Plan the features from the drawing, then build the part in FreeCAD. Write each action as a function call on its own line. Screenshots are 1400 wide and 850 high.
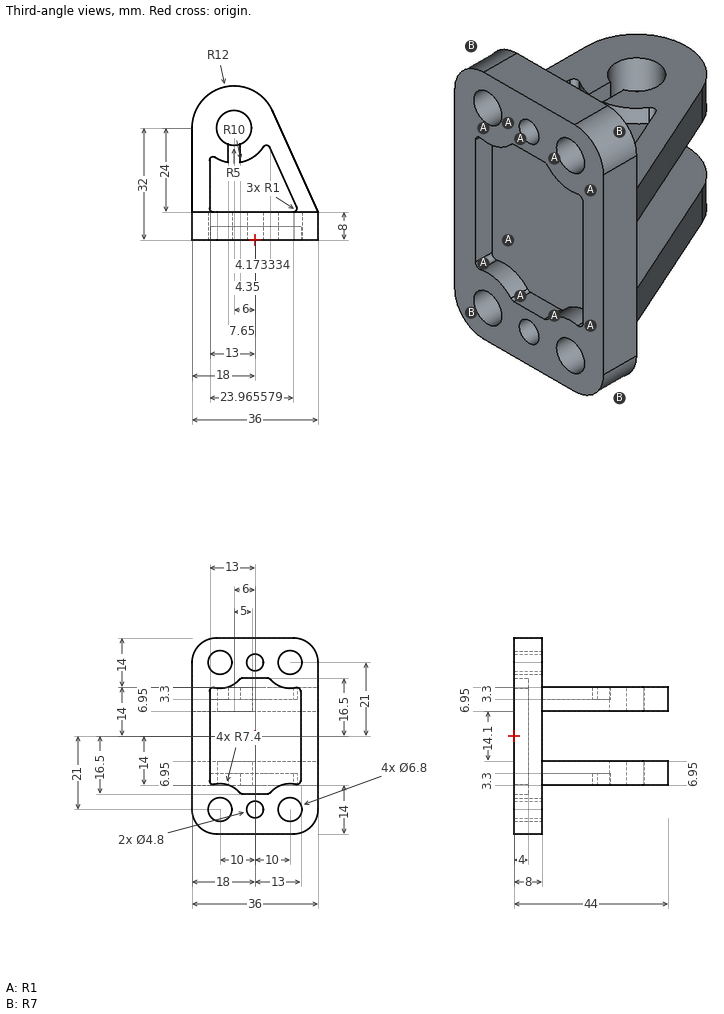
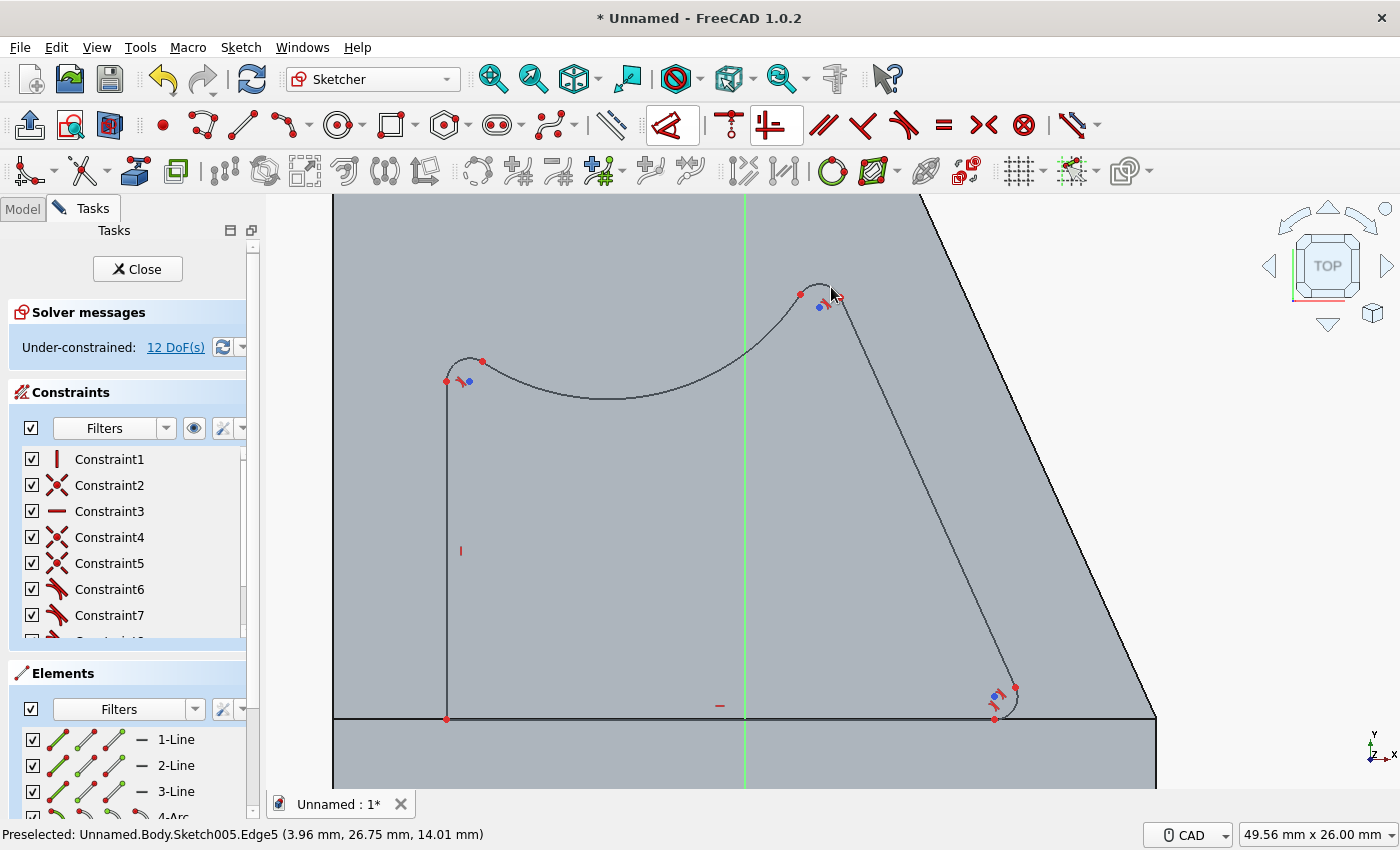
click(831, 287)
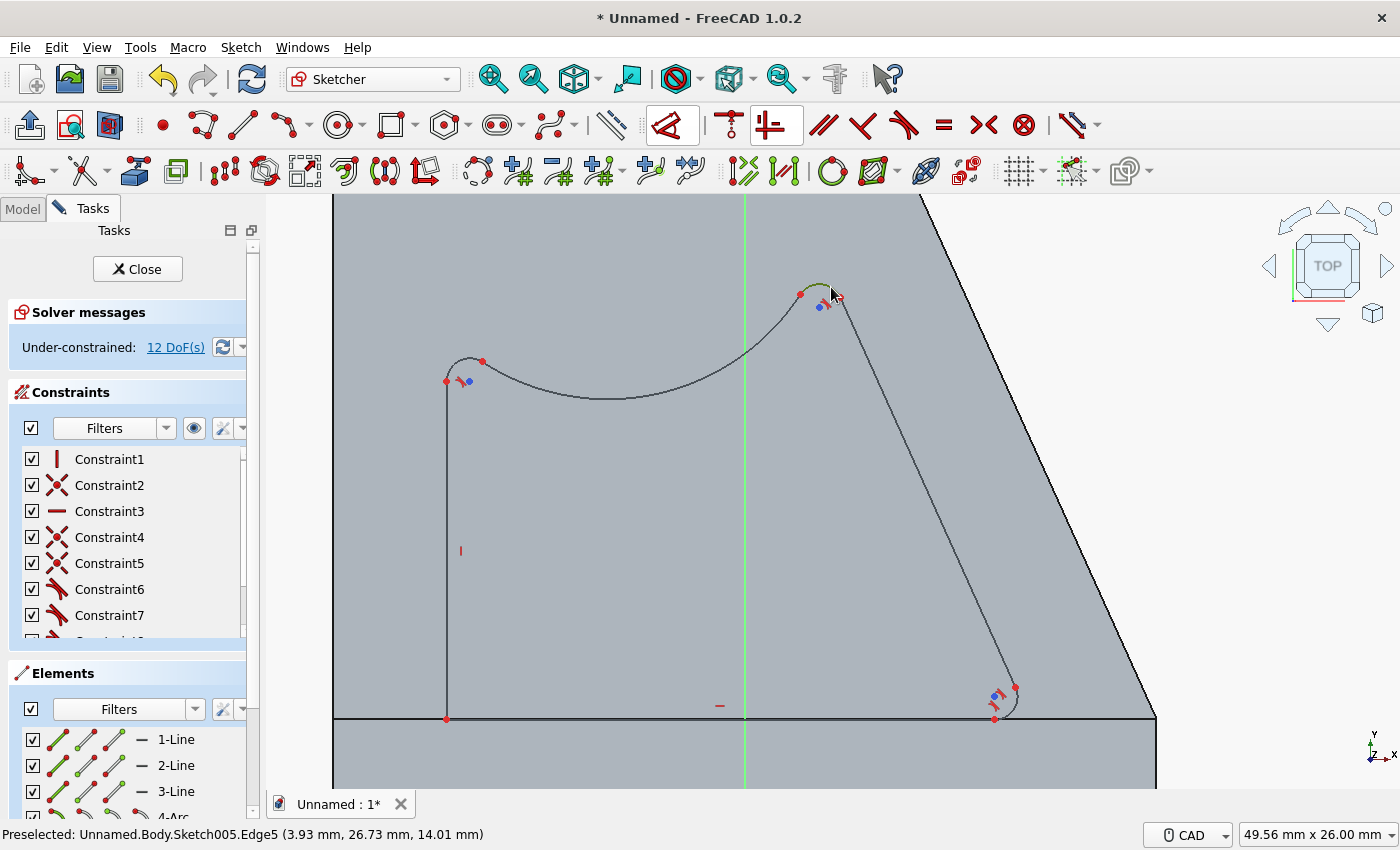
click(583, 398)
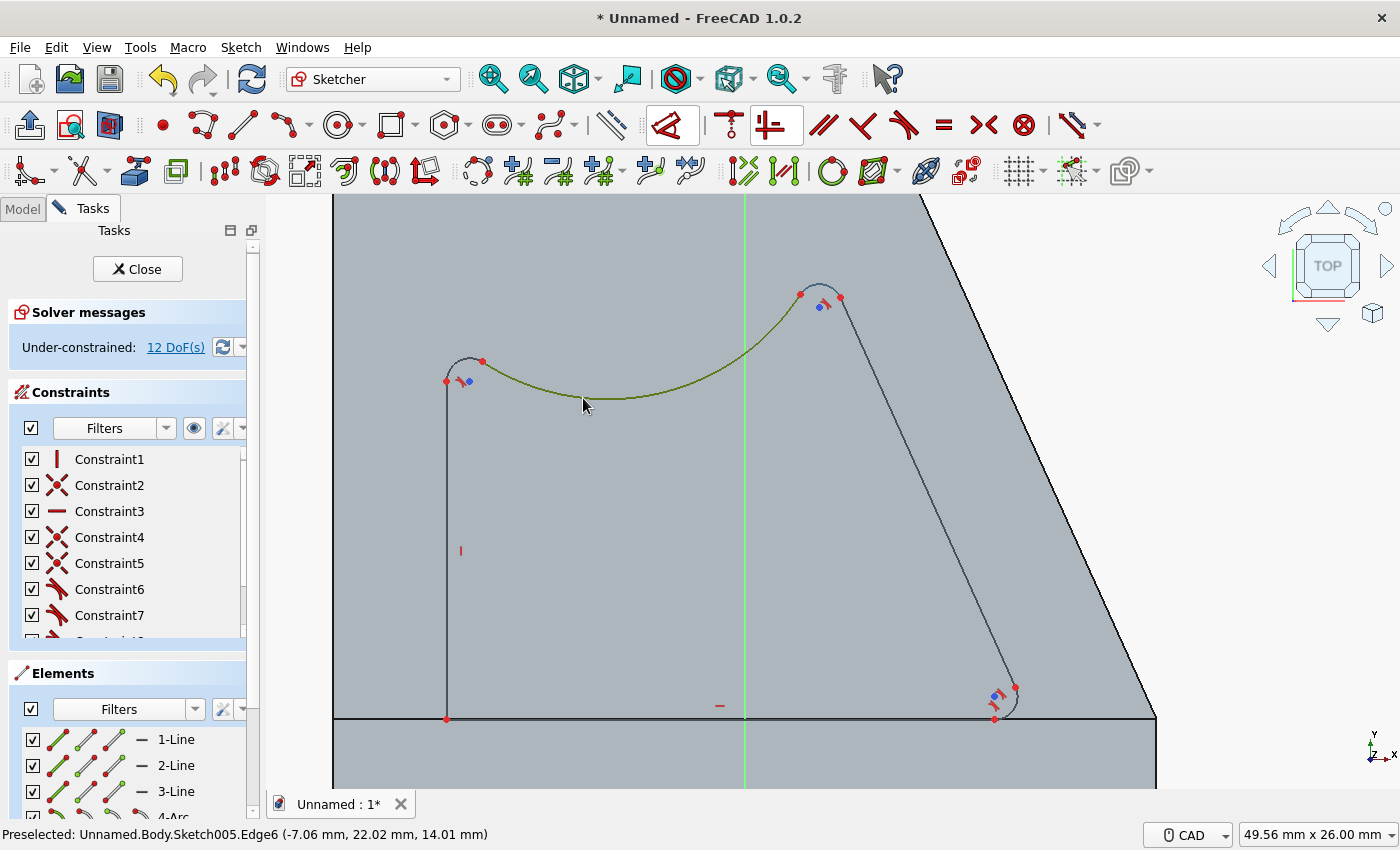
click(904, 126)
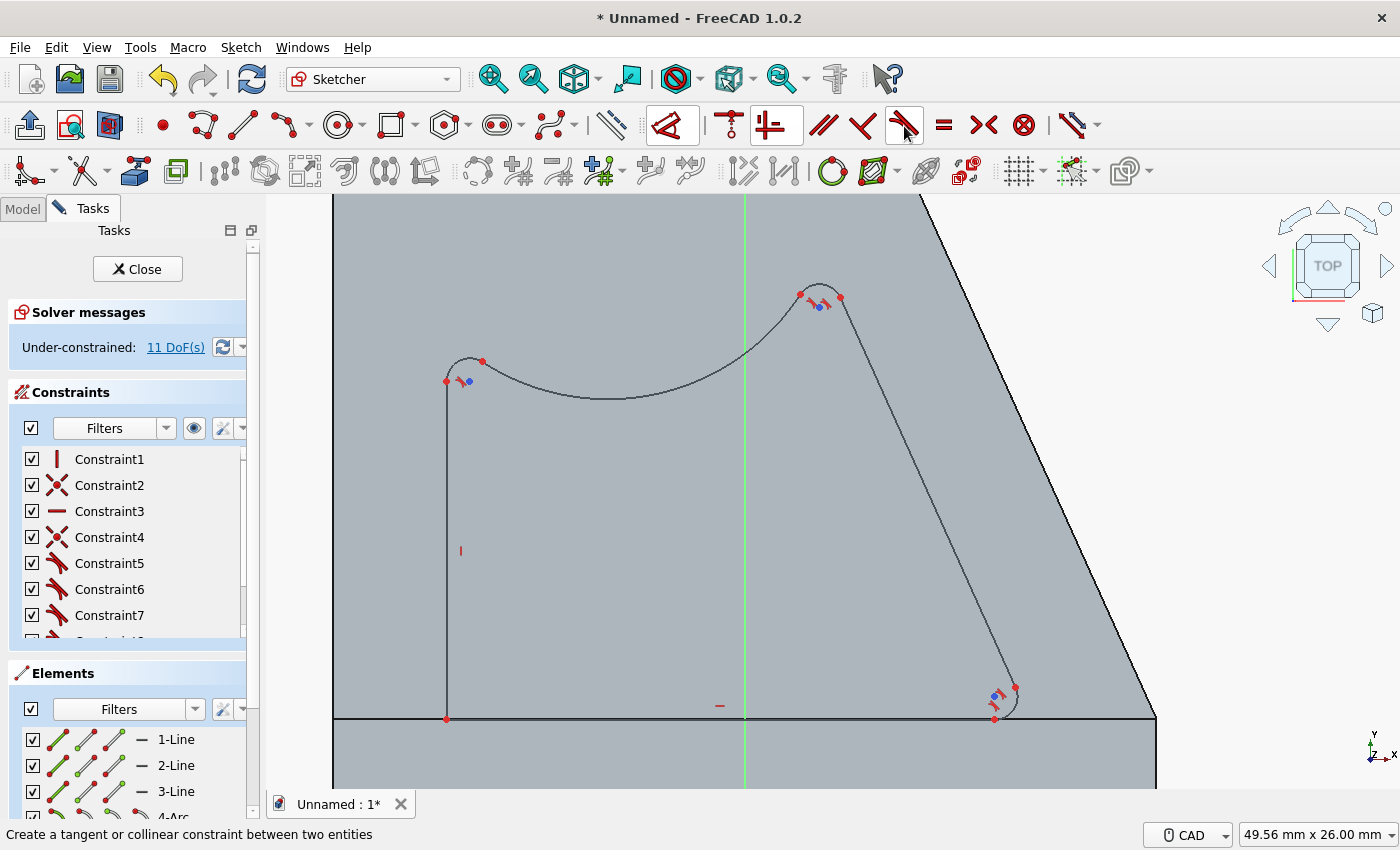
click(583, 398)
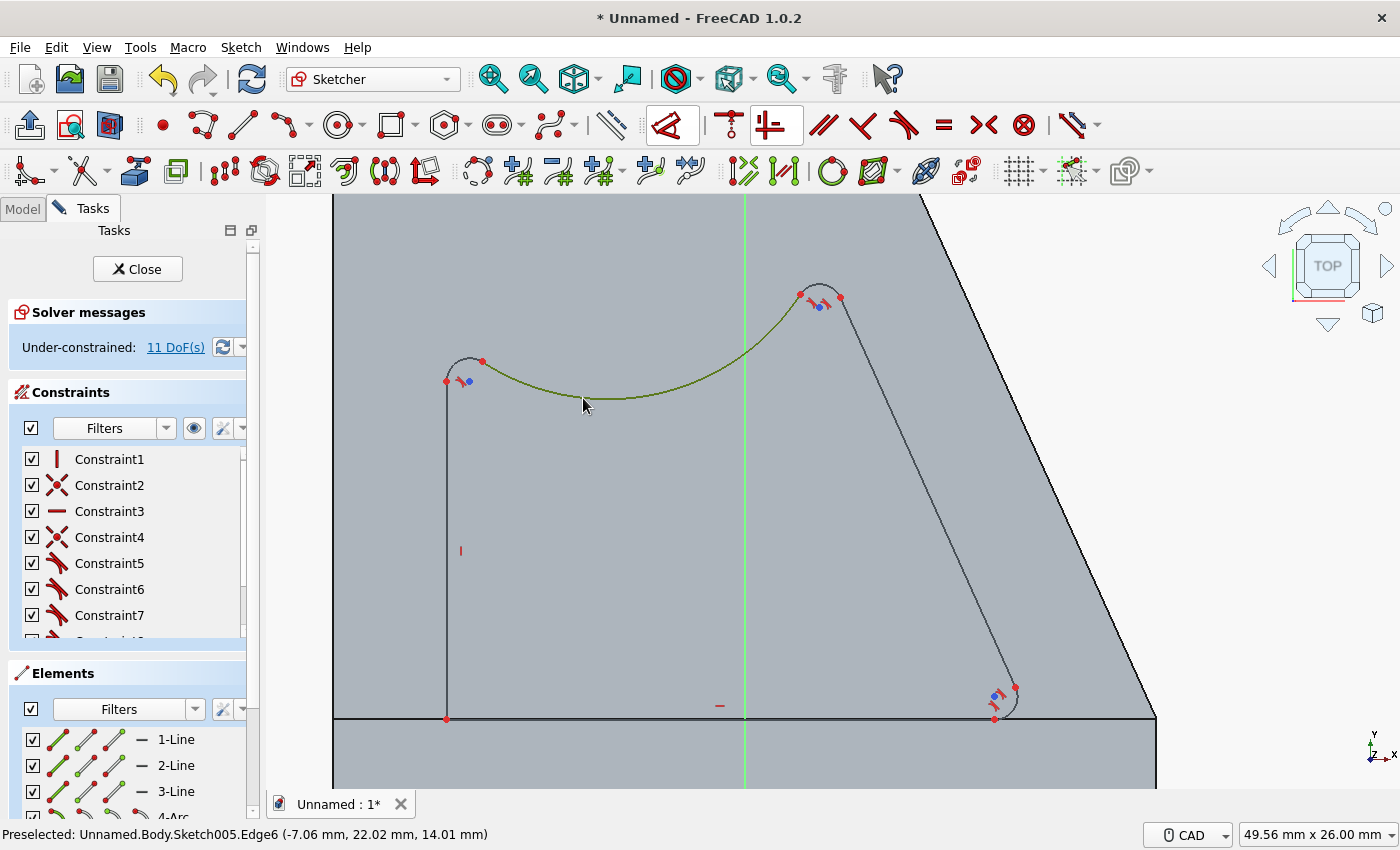
click(468, 358)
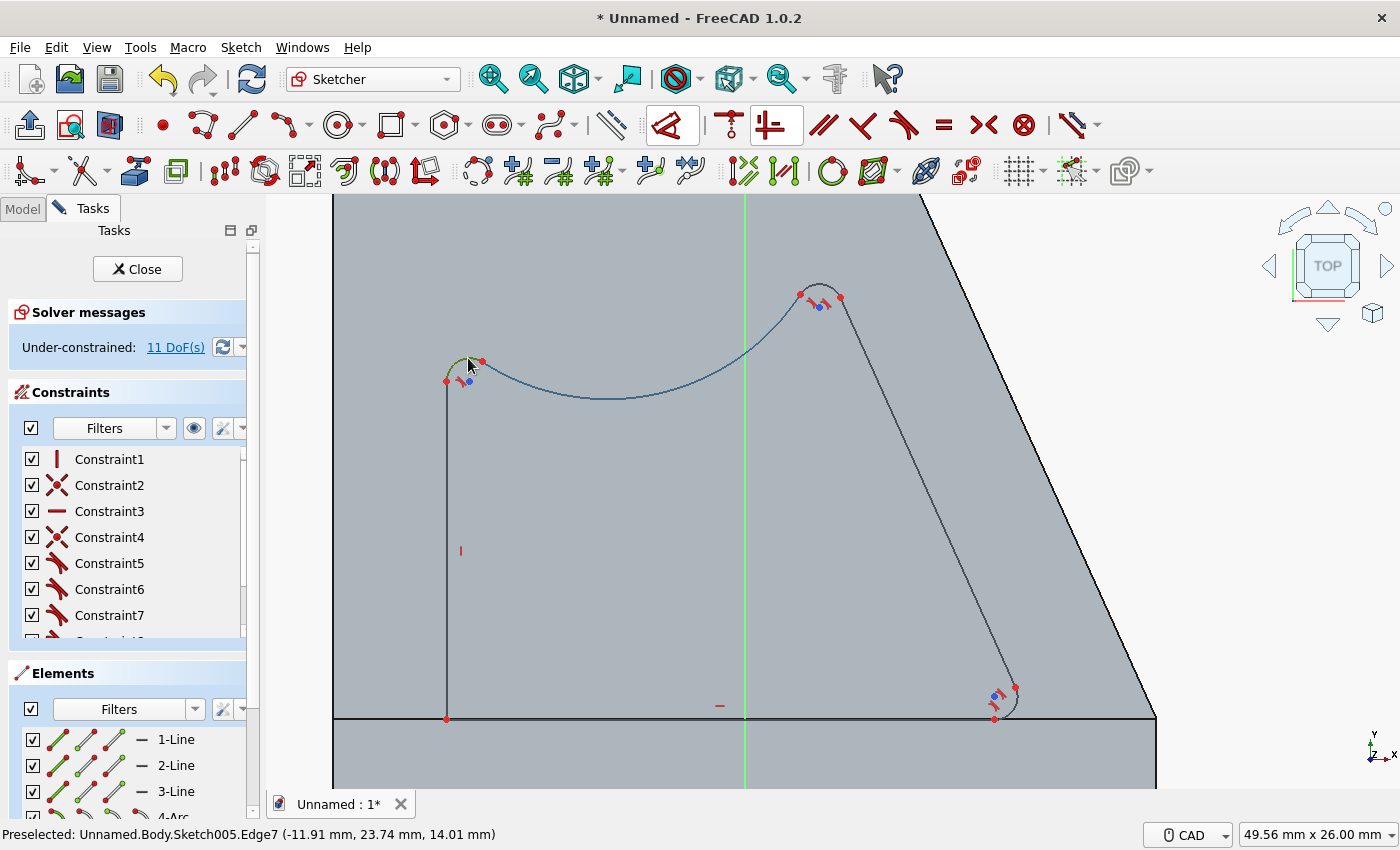
click(904, 126)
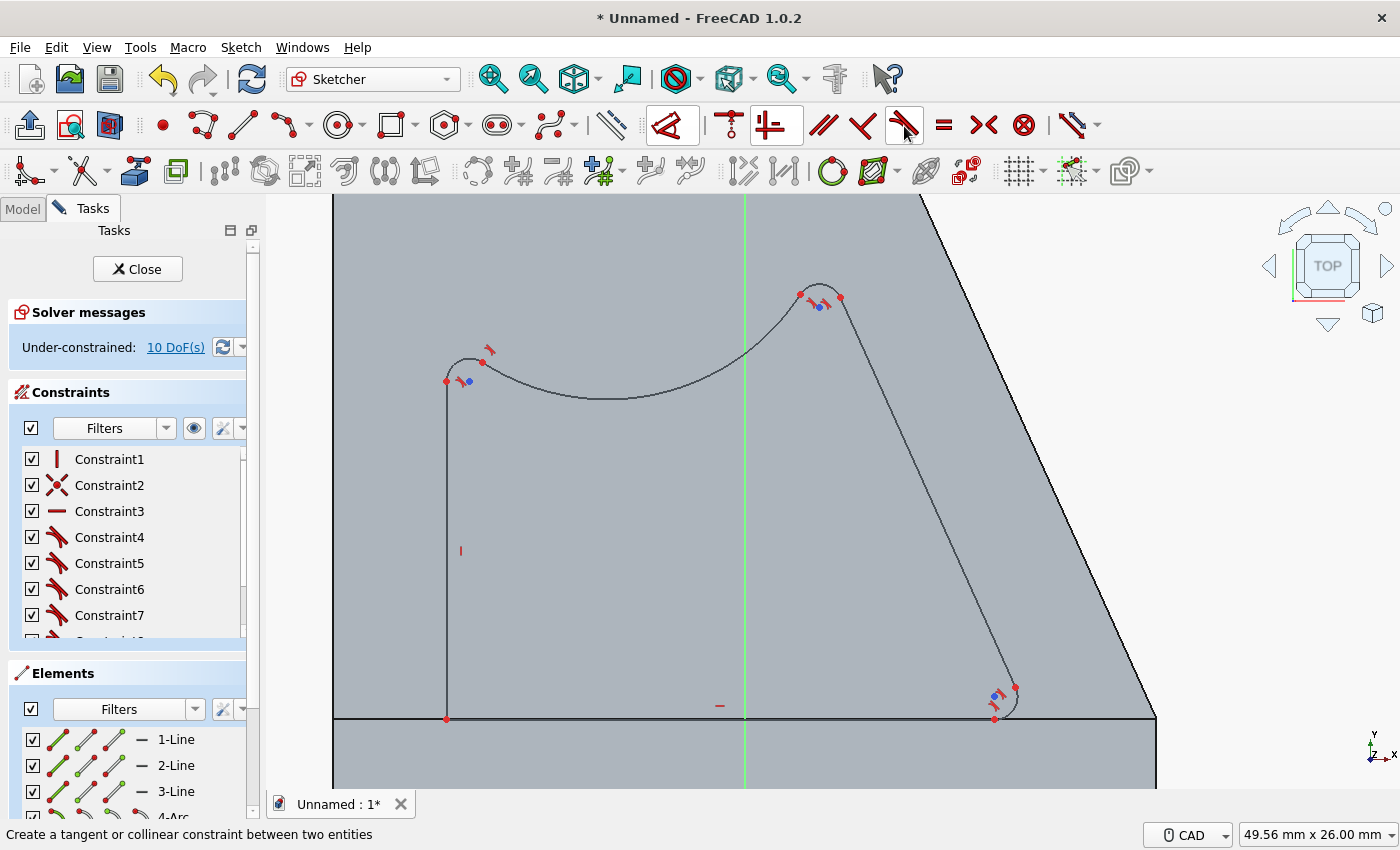
click(1007, 716)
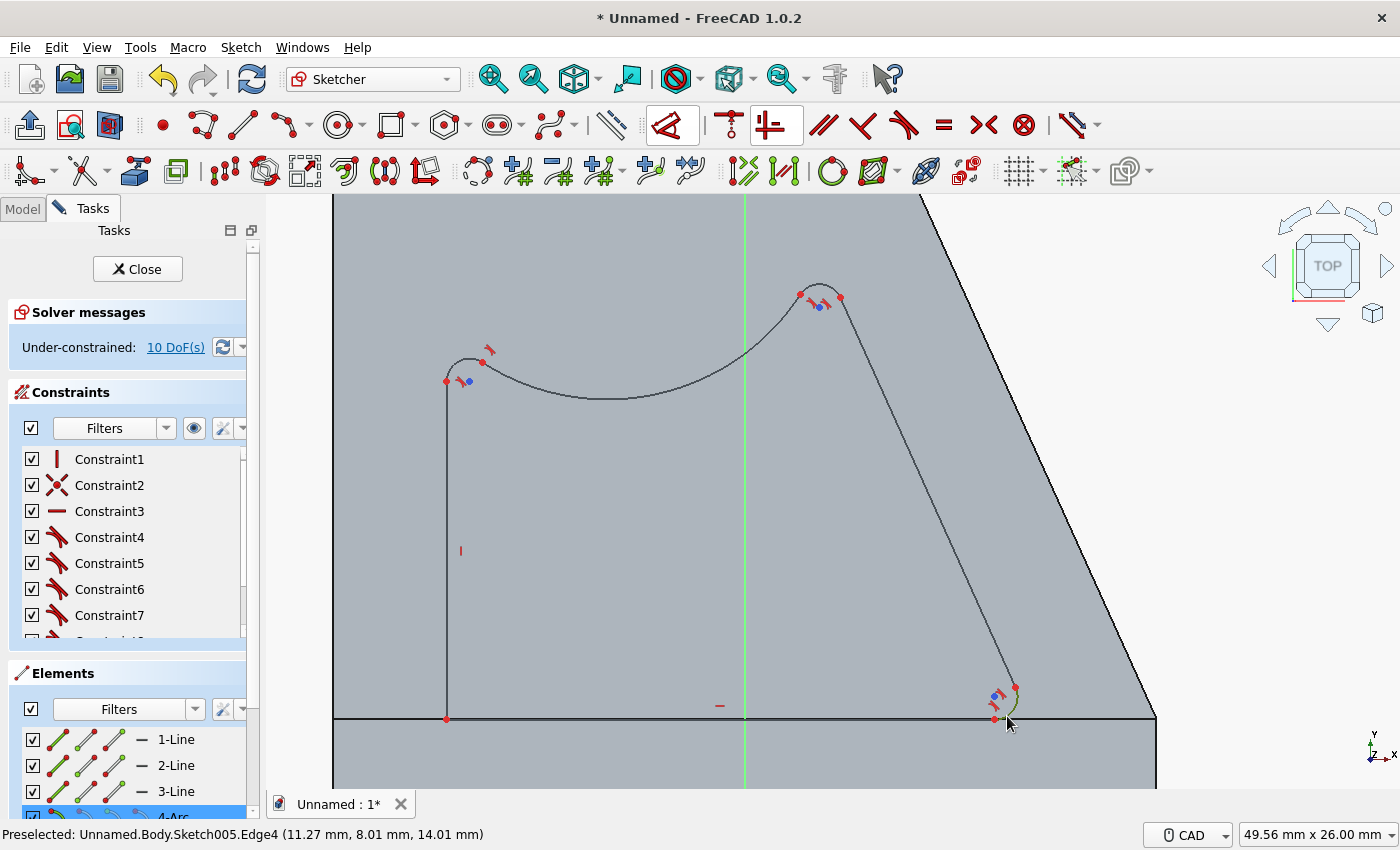
click(831, 287)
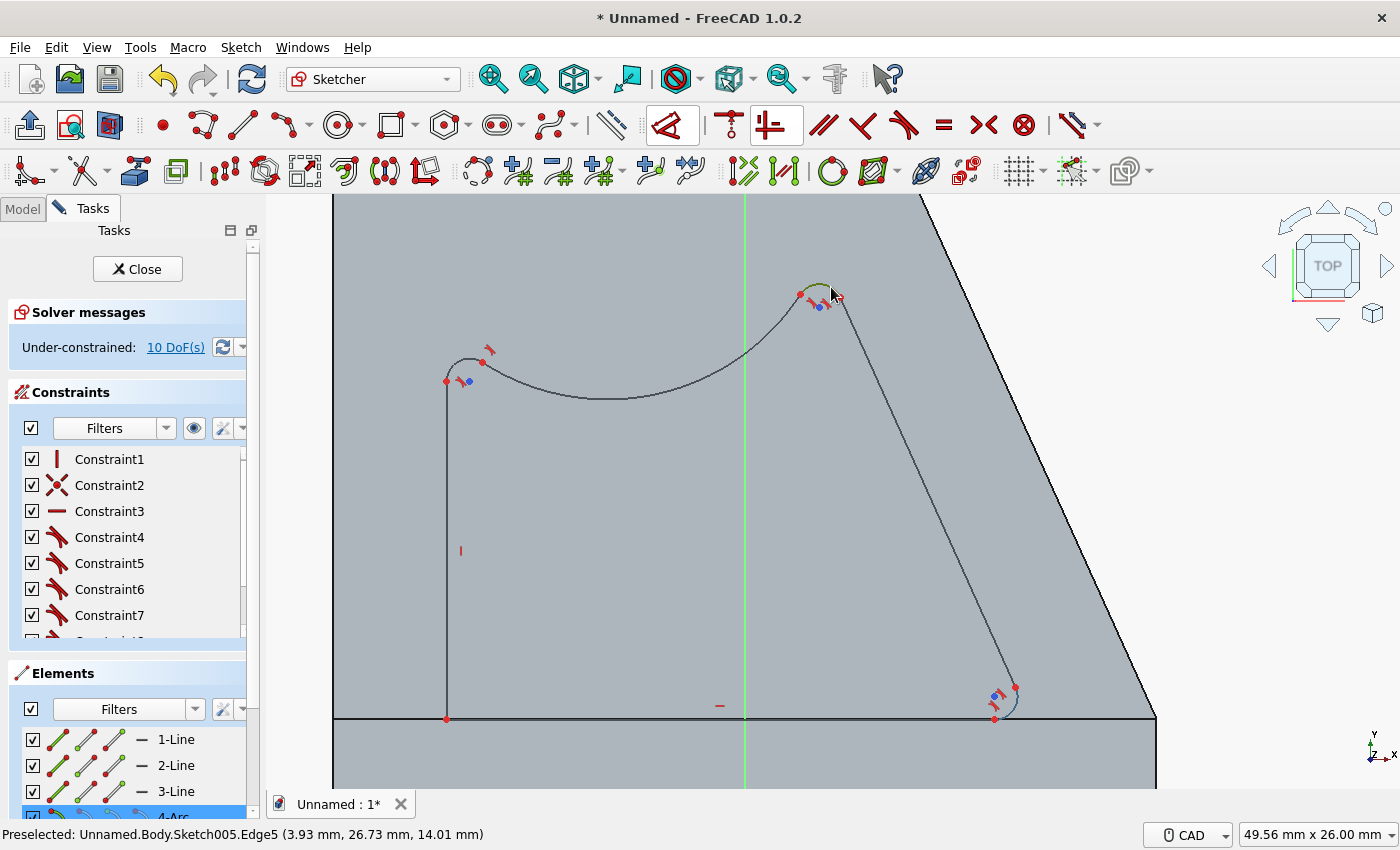
click(468, 359)